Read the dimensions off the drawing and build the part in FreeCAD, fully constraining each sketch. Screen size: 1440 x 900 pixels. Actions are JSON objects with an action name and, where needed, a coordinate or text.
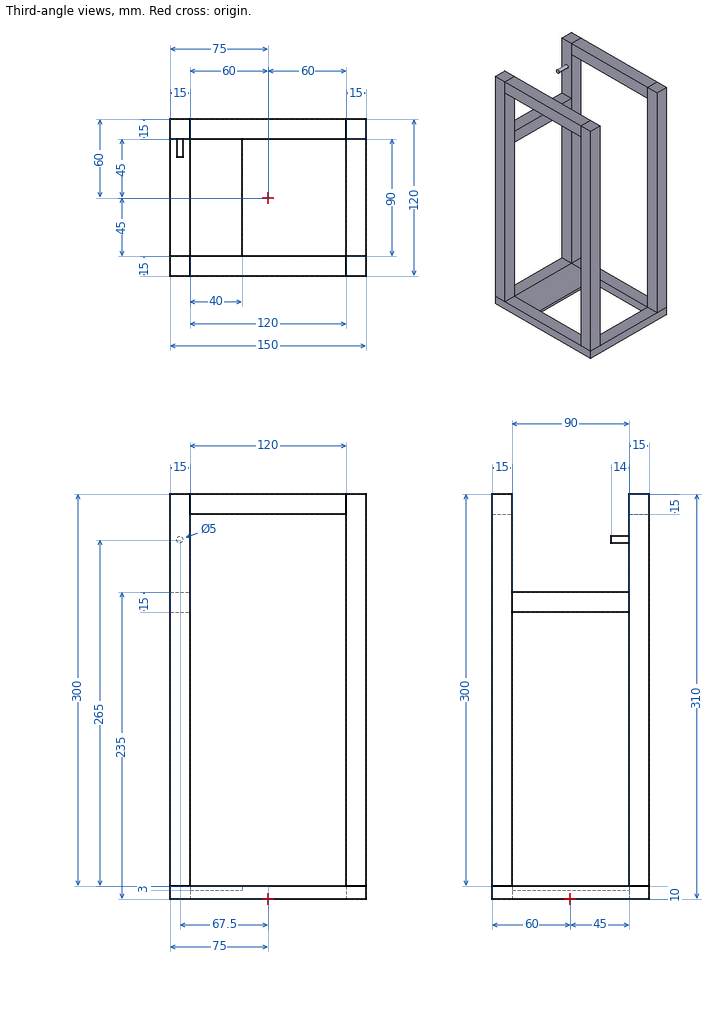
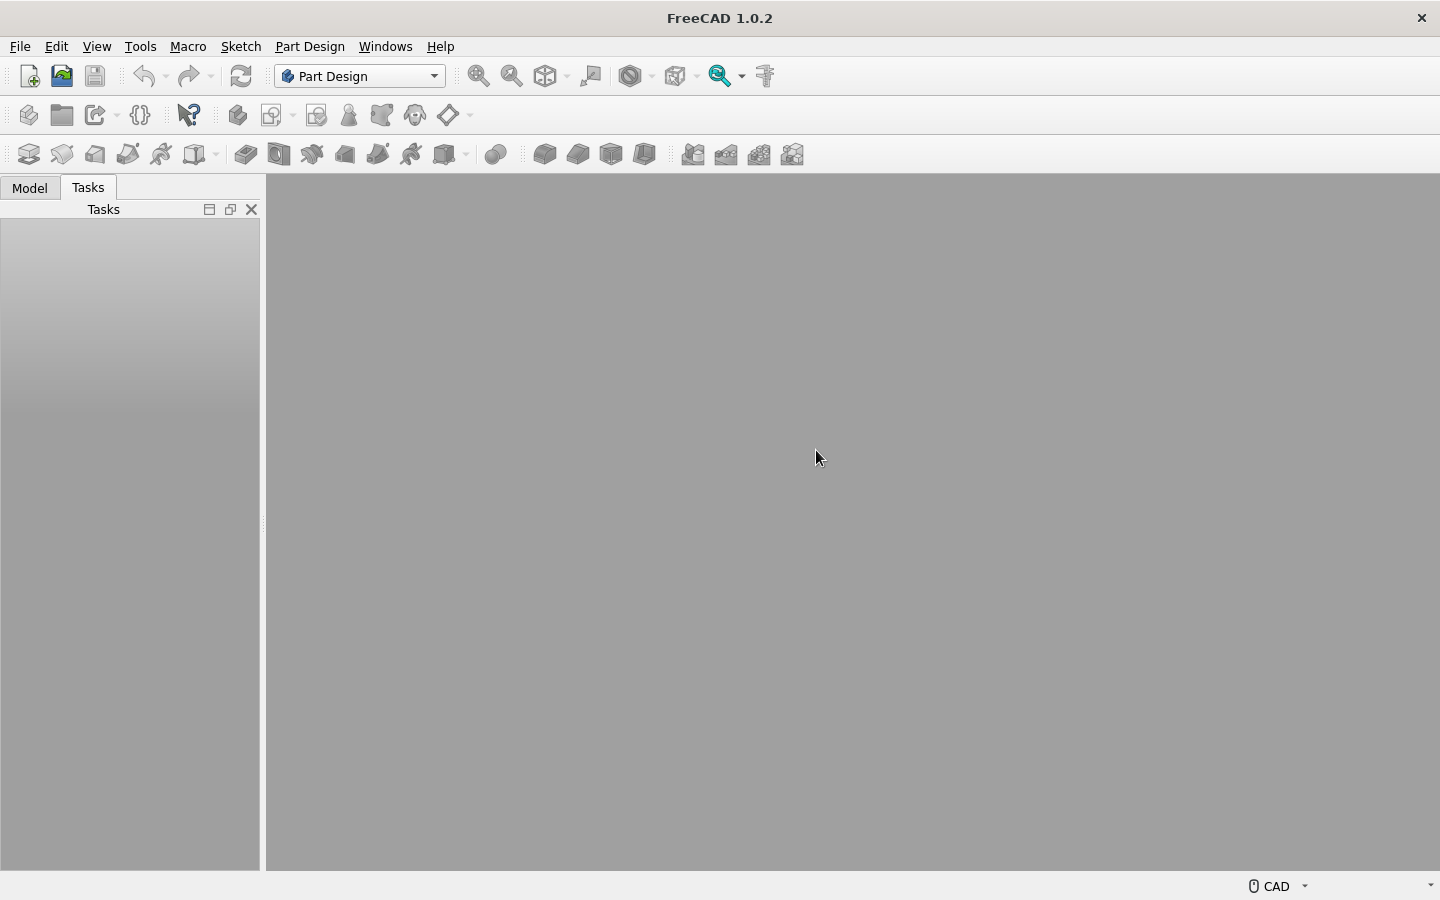
{"action": "left_click", "coordinate": [29, 76]}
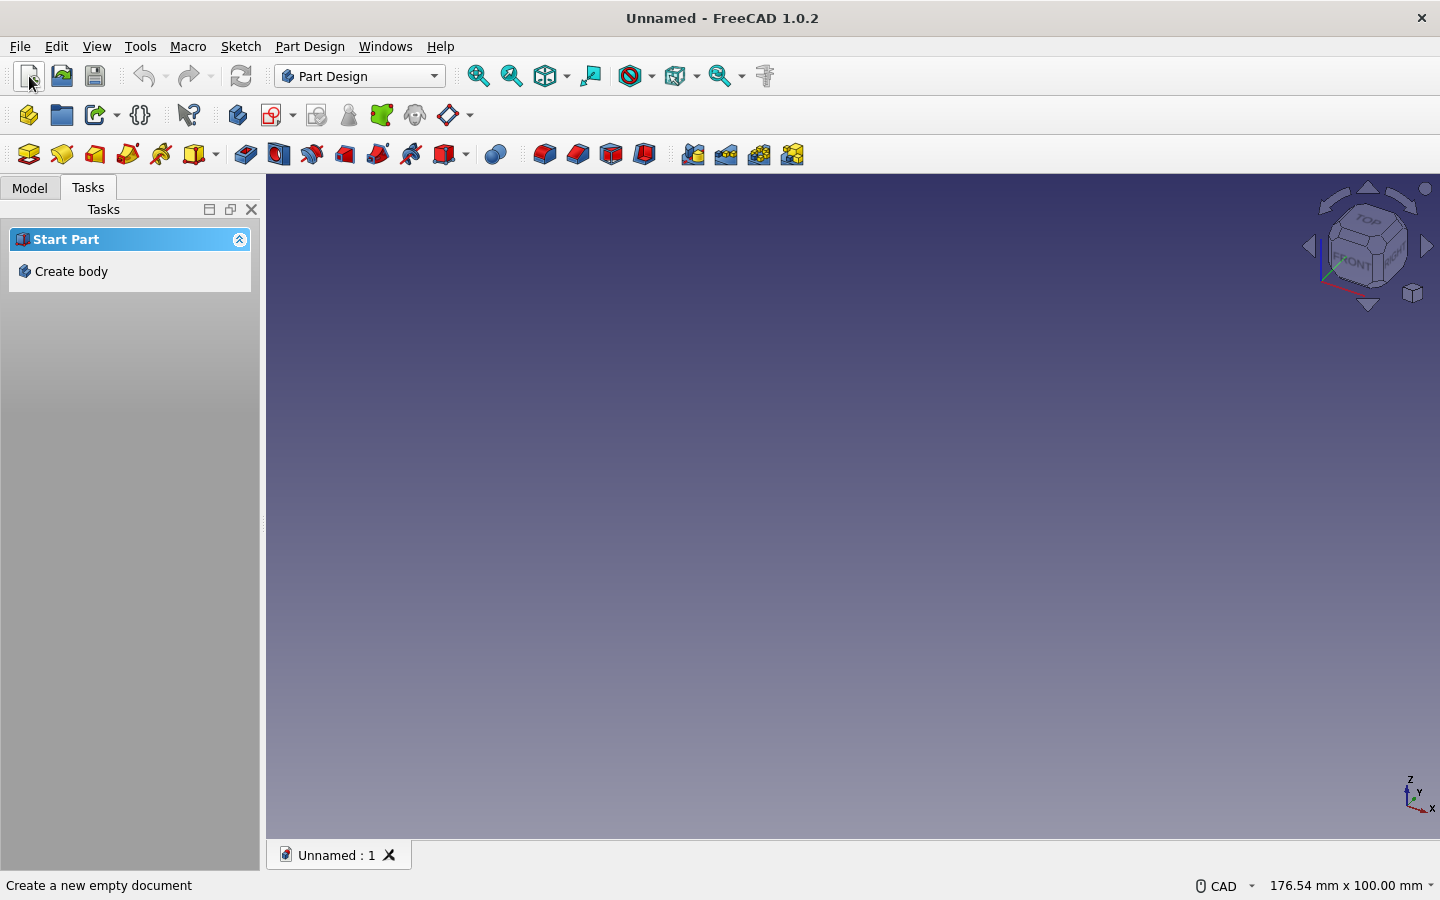
{"action": "left_click", "coordinate": [270, 116]}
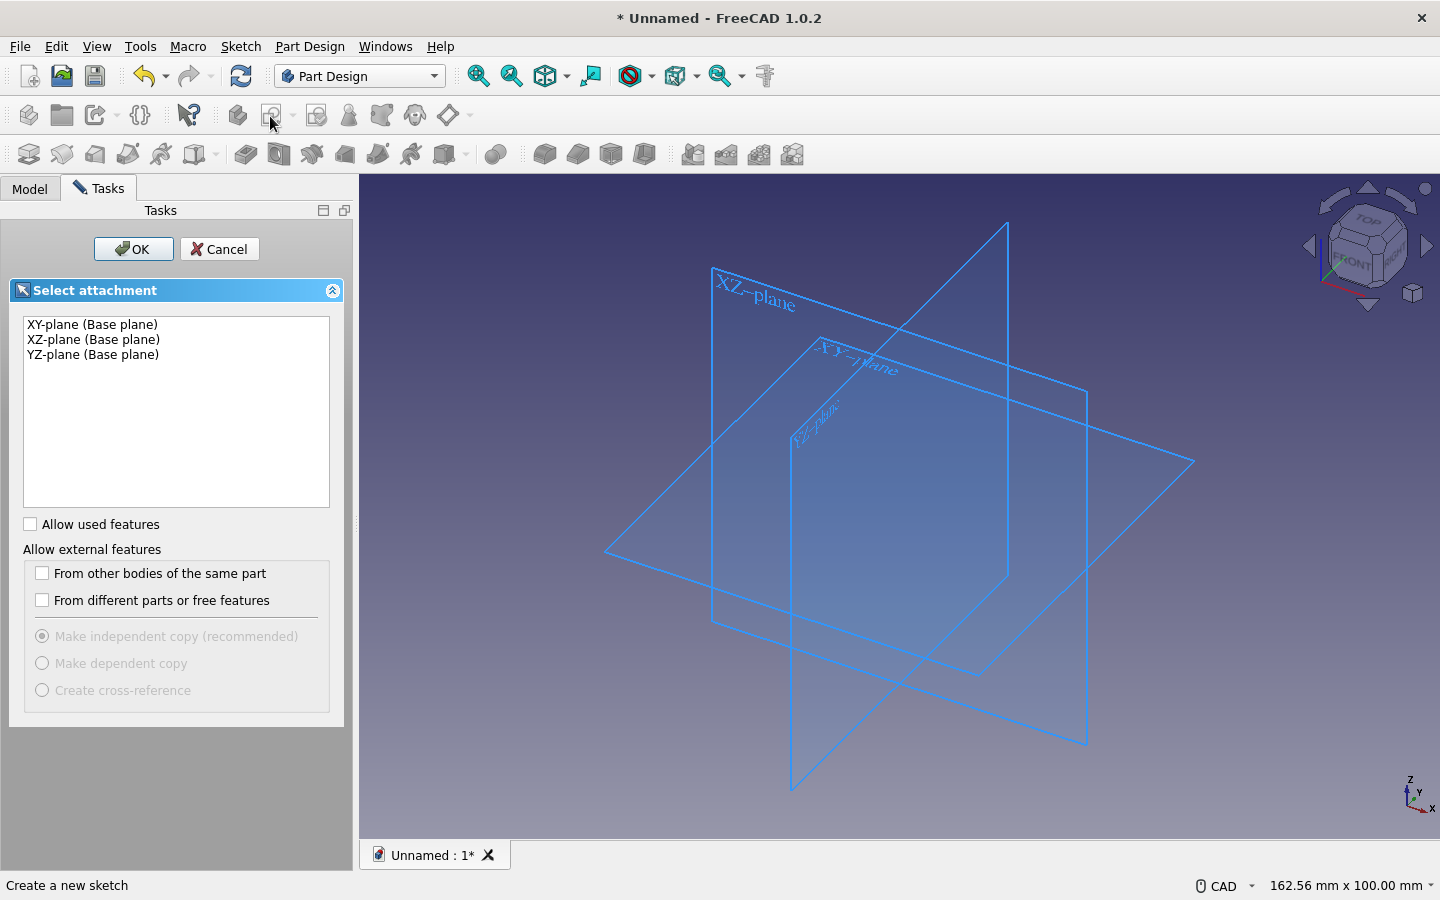
{"action": "left_click", "coordinate": [84, 324]}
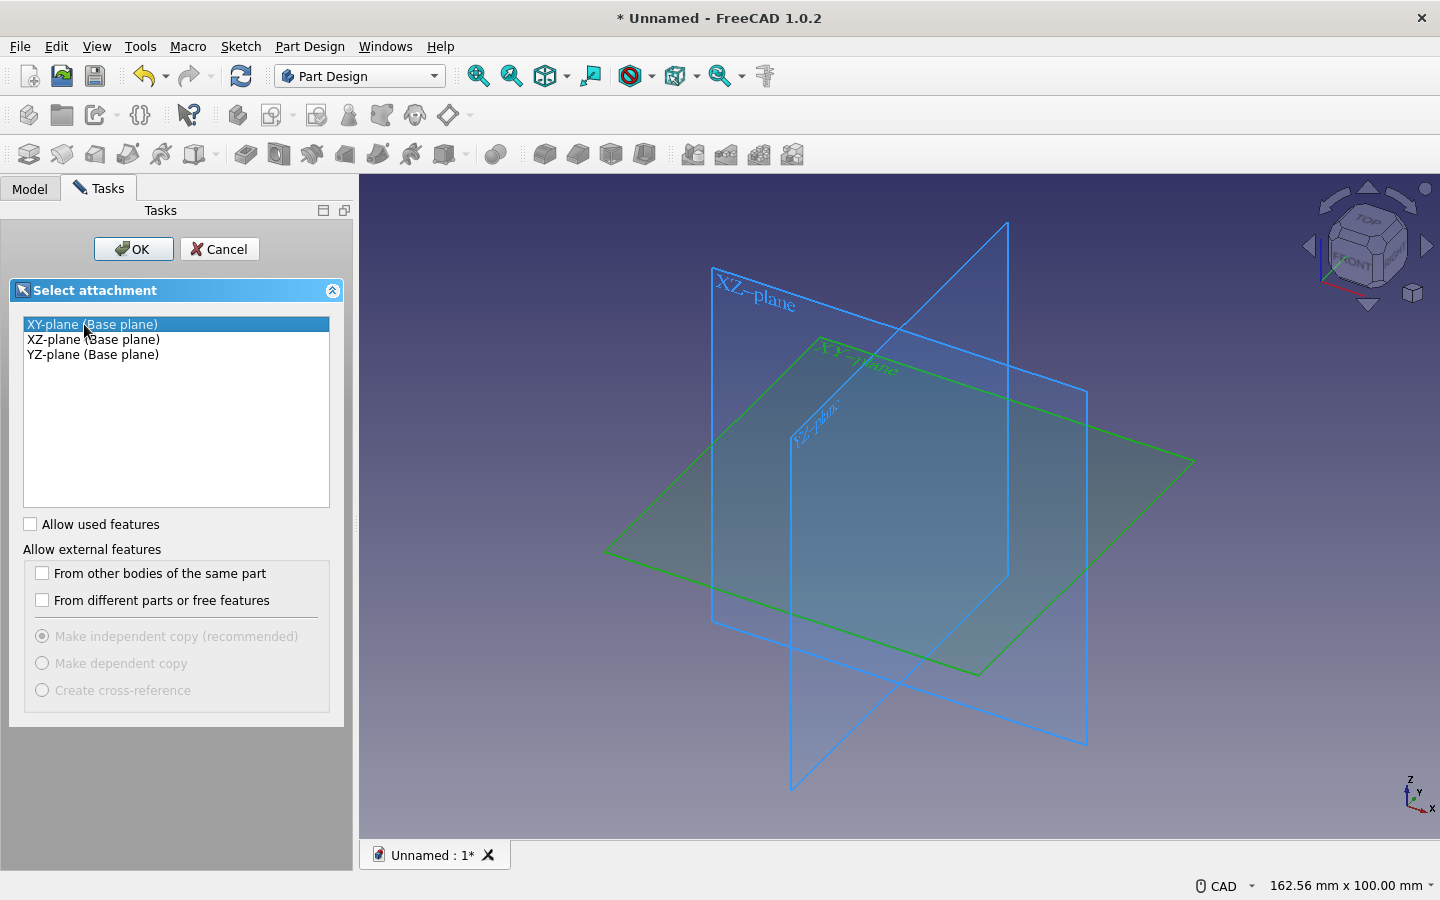
{"action": "left_click", "coordinate": [134, 249]}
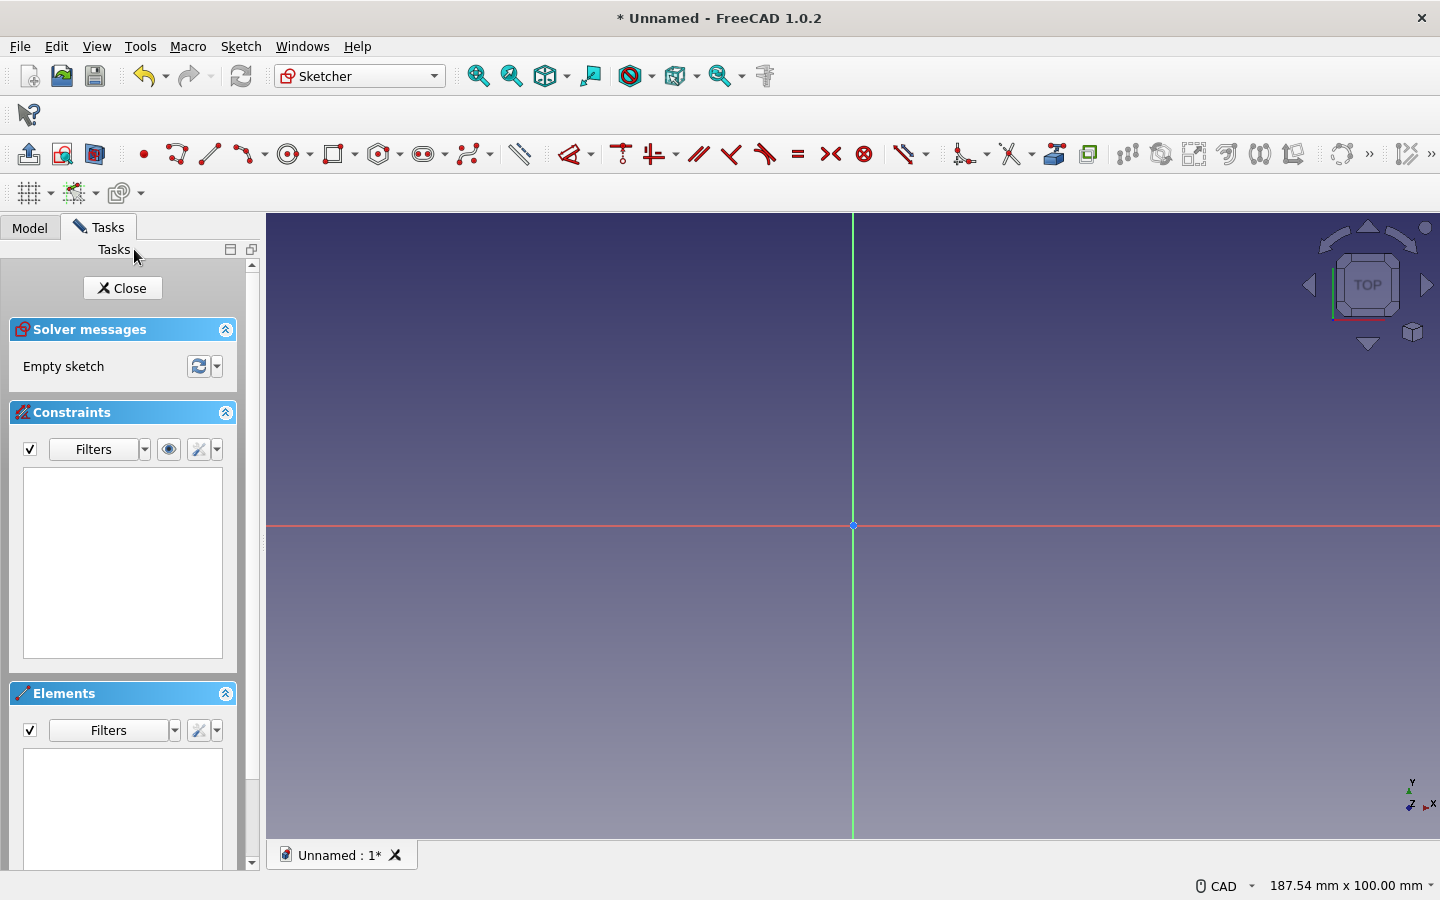
{"action": "scroll", "coordinate": [701, 526], "scroll_direction": "down", "scroll_amount": 3}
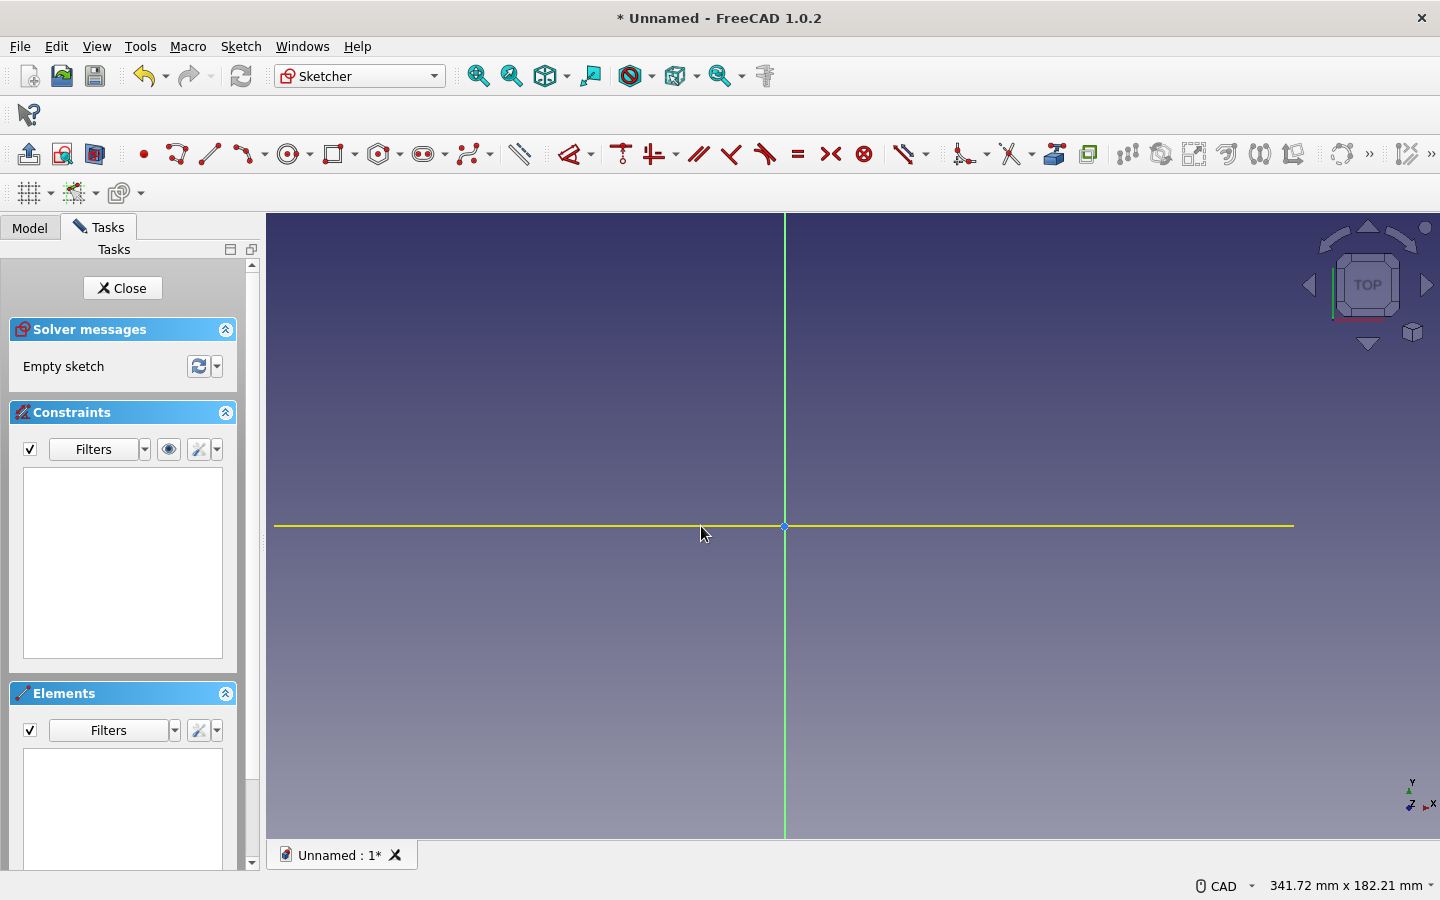
{"action": "left_click", "coordinate": [354, 154]}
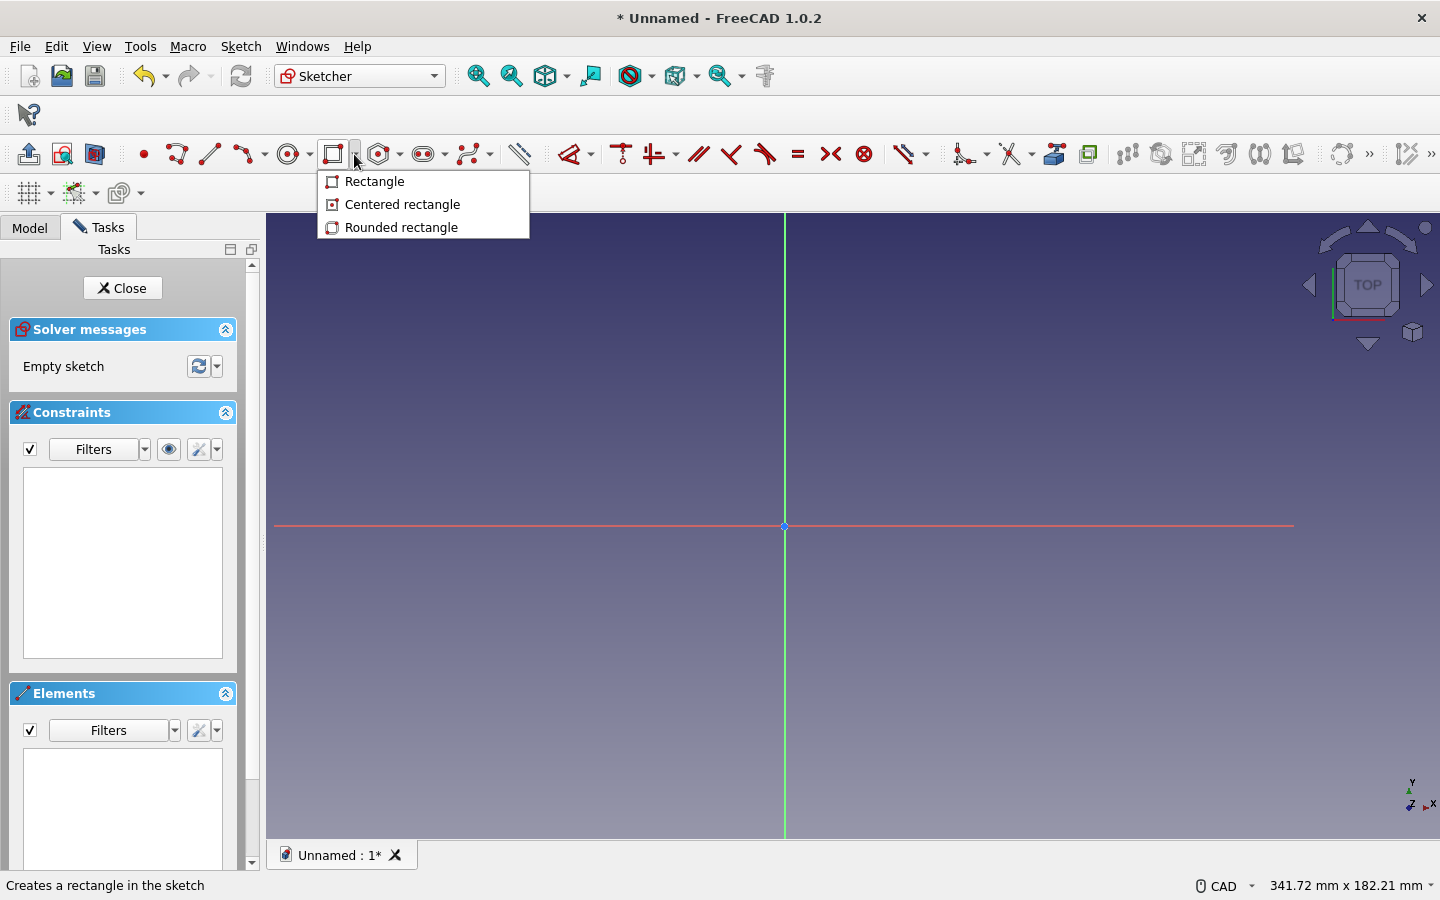
{"action": "left_click", "coordinate": [424, 204]}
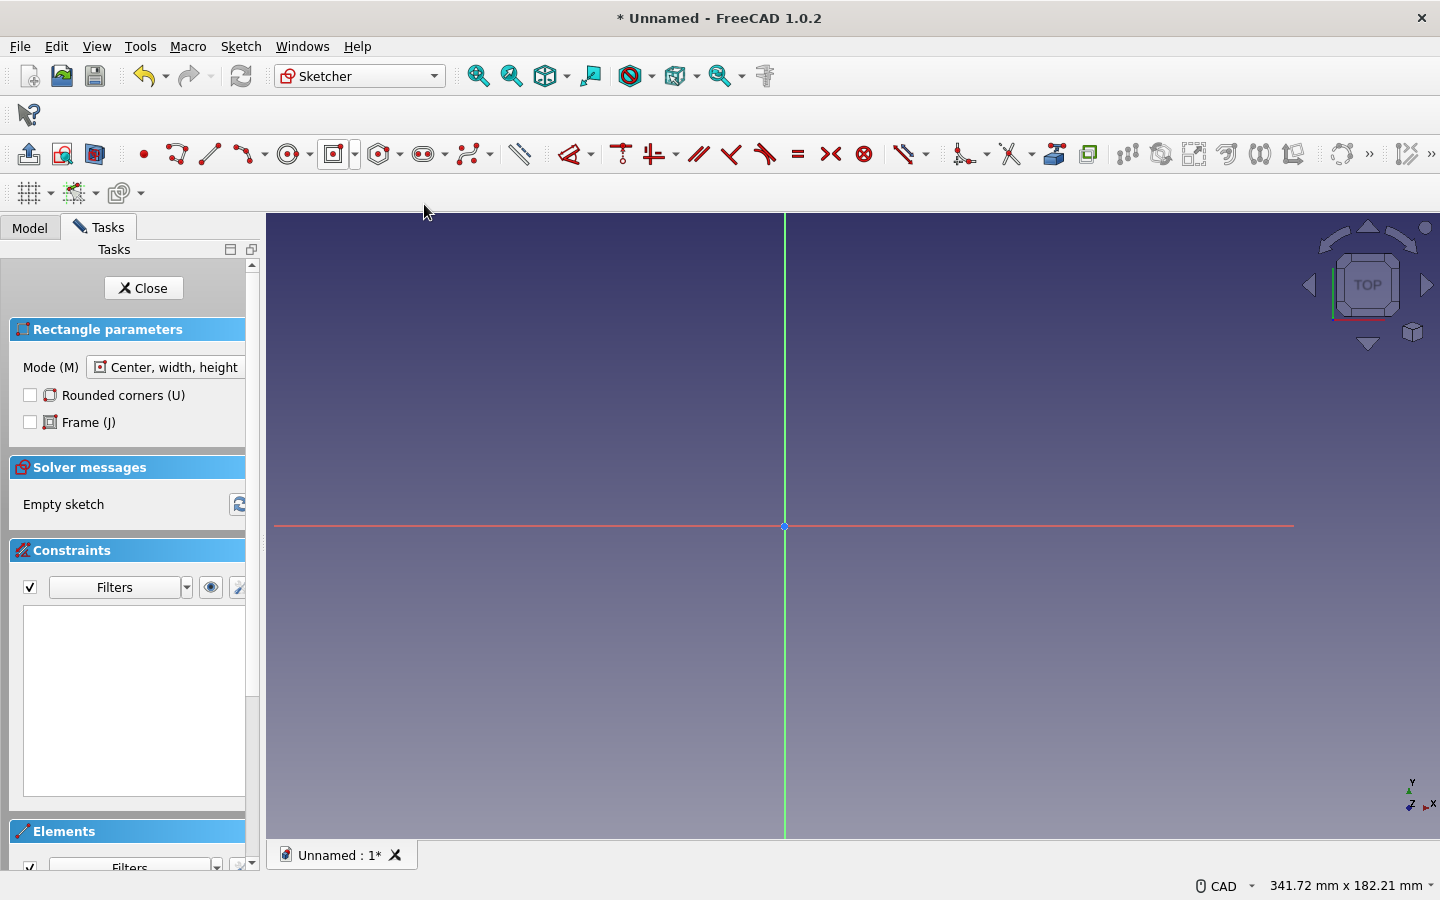
{"action": "left_click", "coordinate": [785, 526]}
{"action": "left_click", "coordinate": [1042, 320]}
{"action": "key", "text": "Escape"}